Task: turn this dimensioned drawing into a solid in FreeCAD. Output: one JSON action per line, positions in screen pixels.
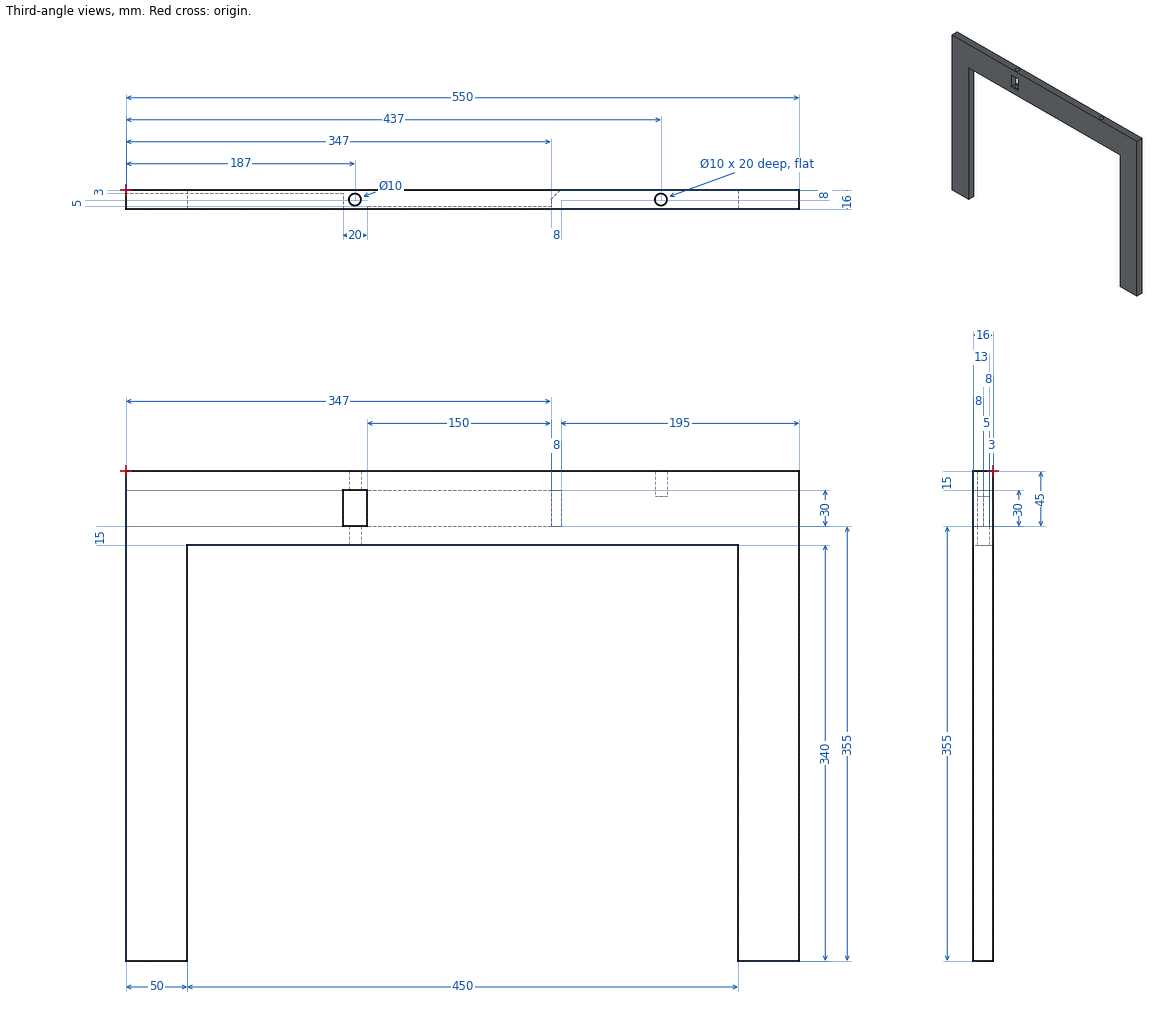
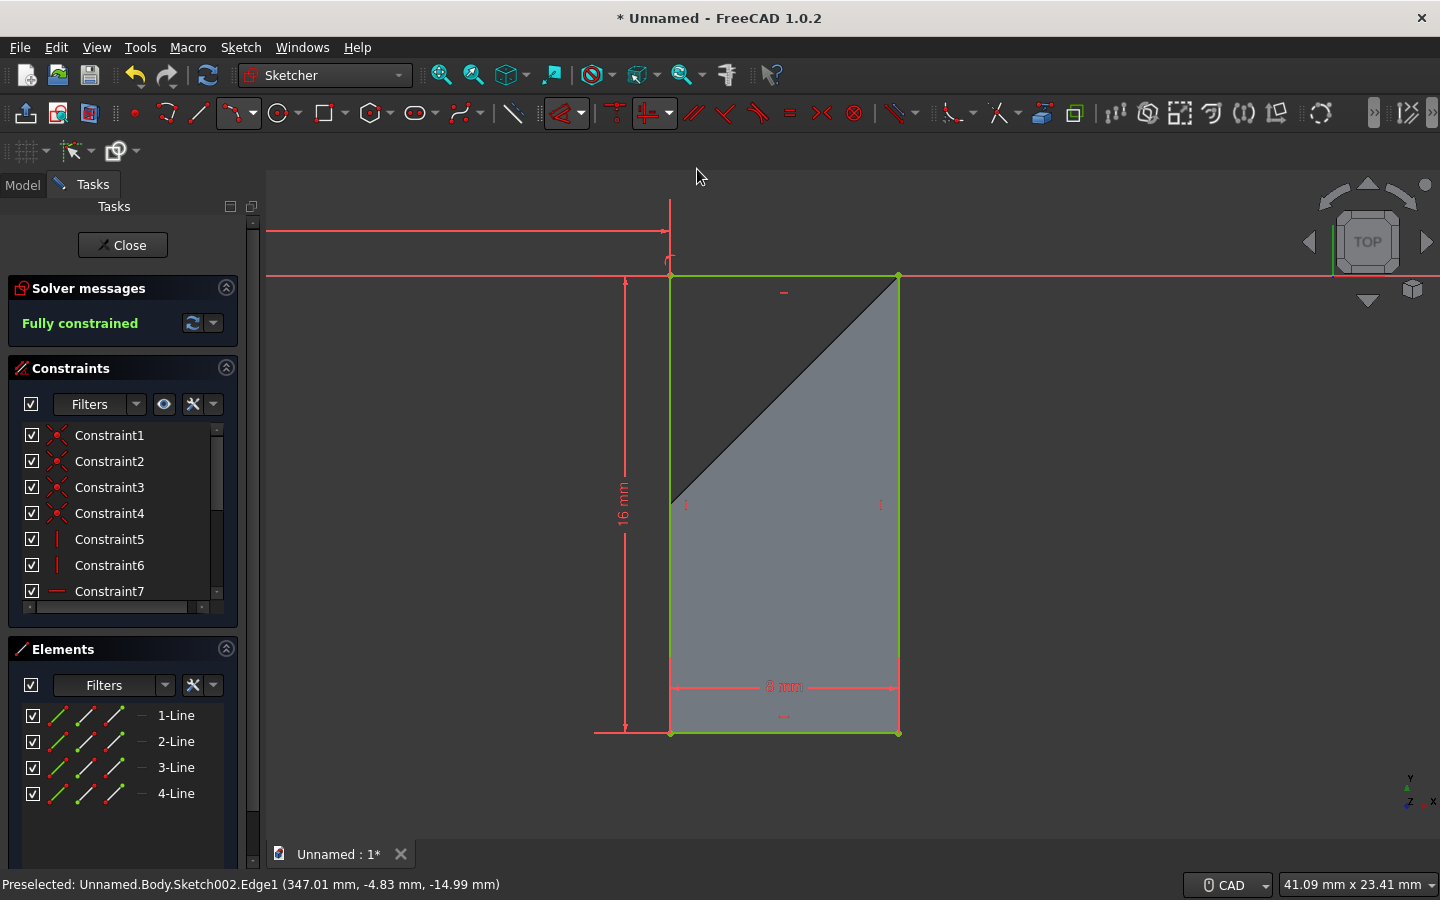
{"action": "left_click", "coordinate": [123, 245]}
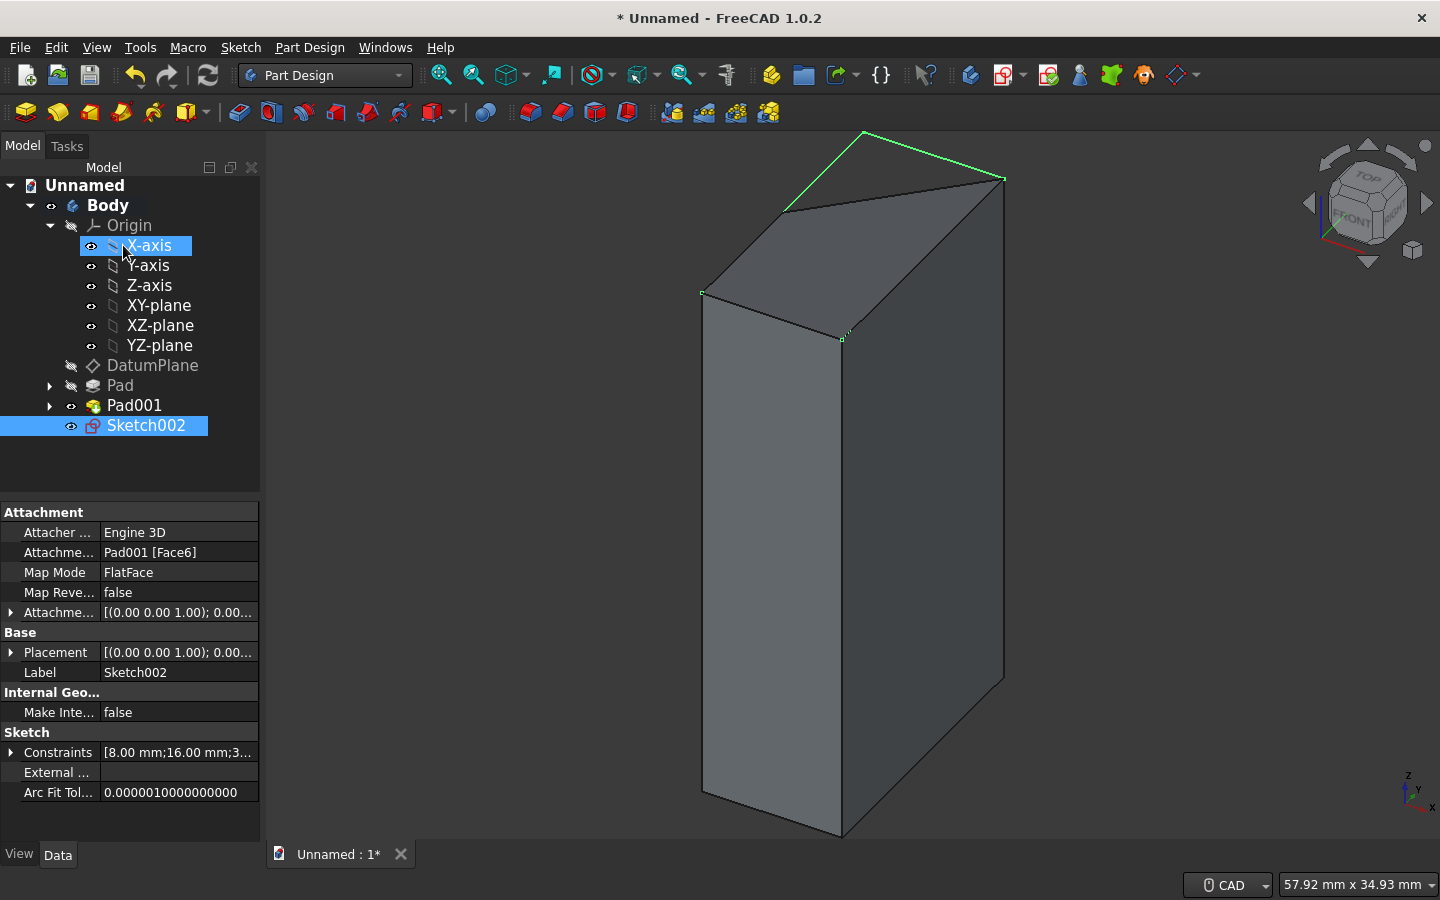
{"action": "left_click", "coordinate": [26, 112]}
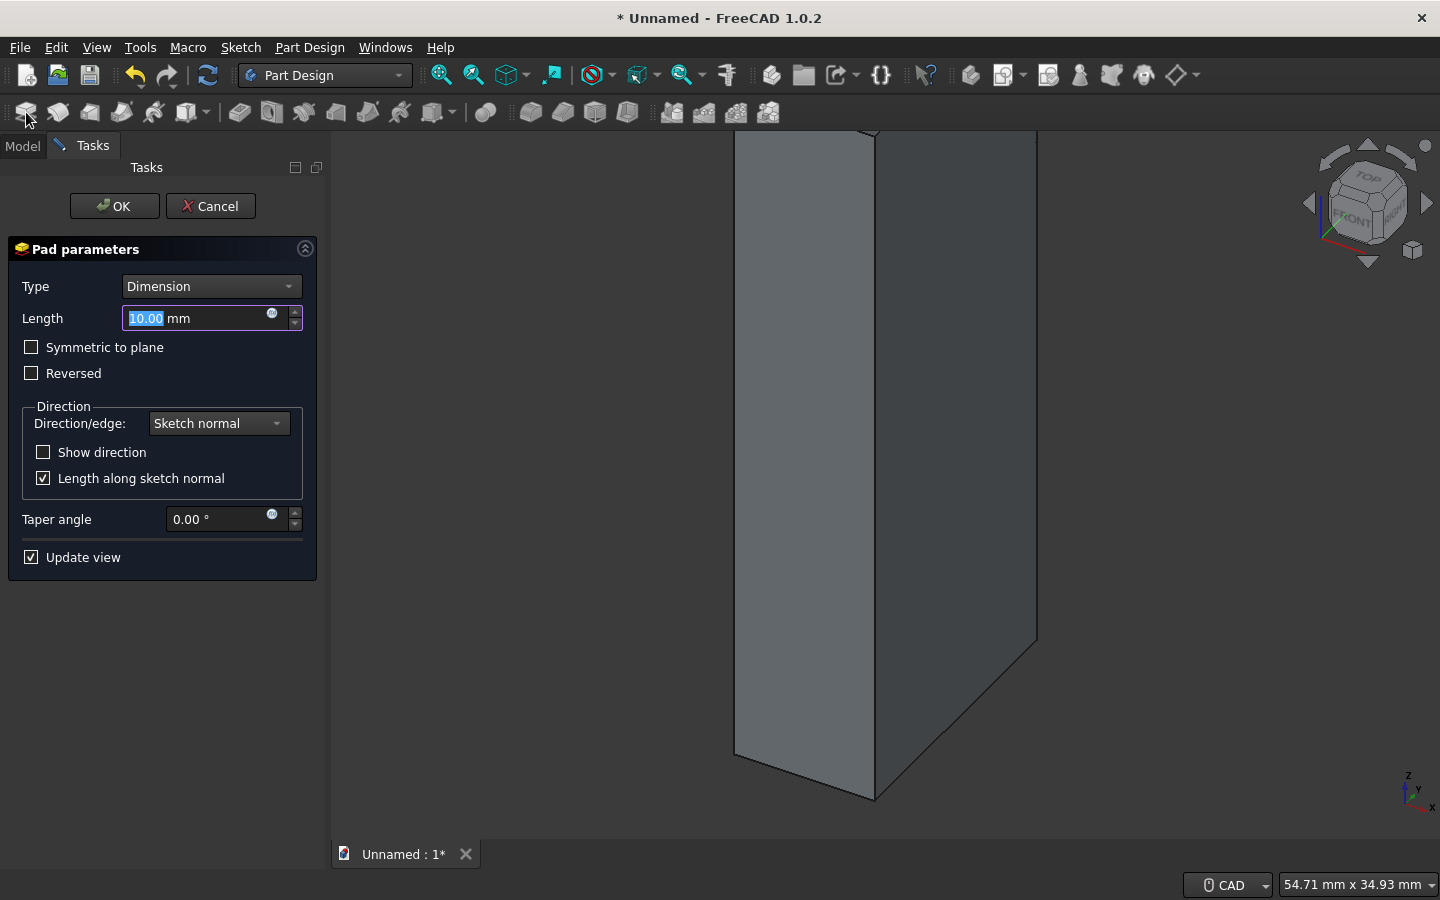
{"action": "type", "text": "15"}
{"action": "key", "text": "Tab"}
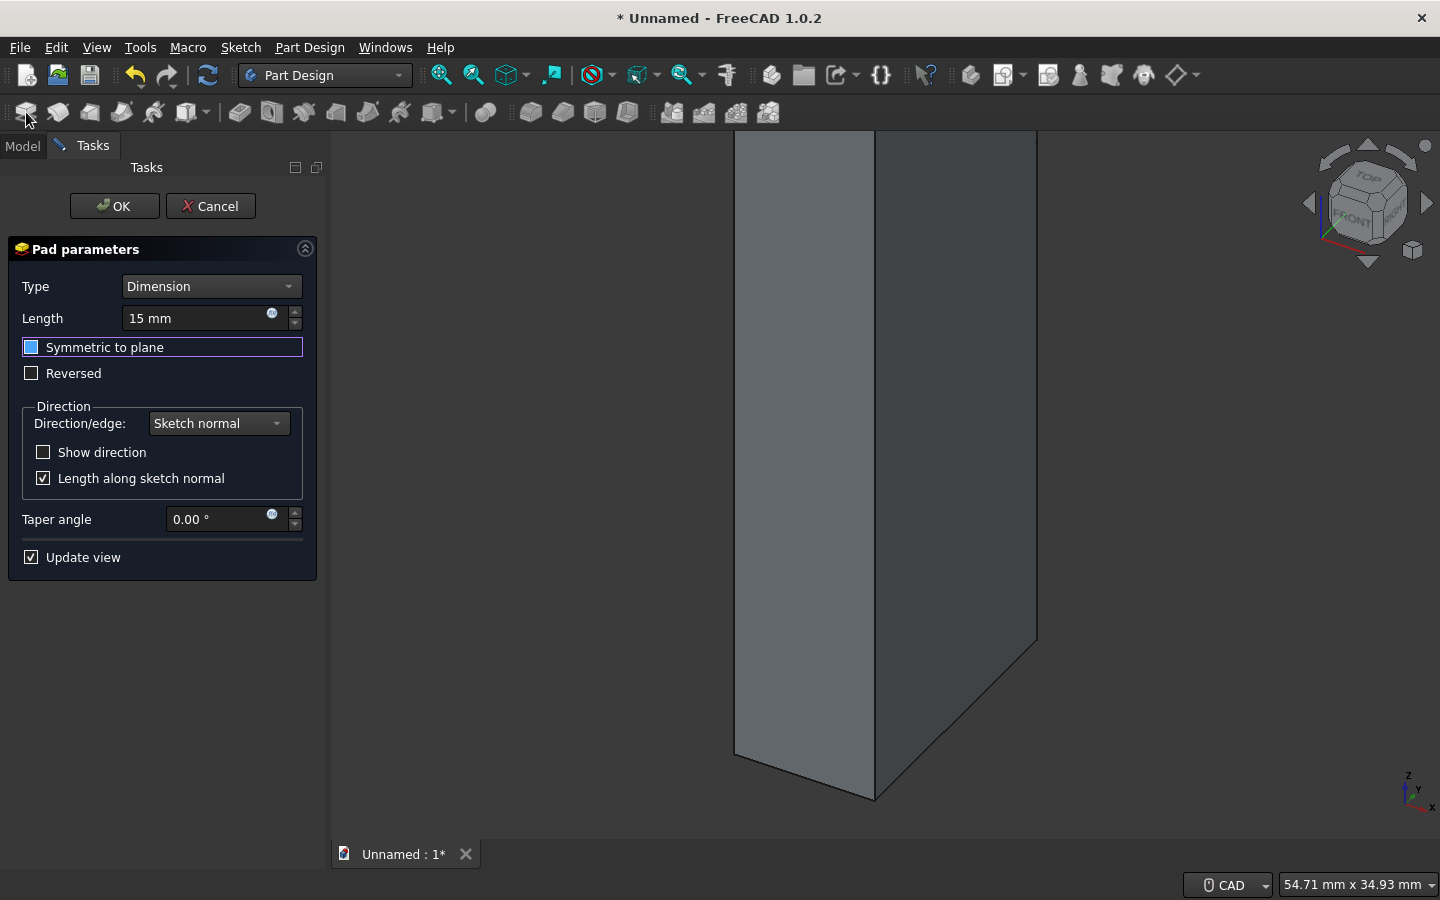
{"action": "left_click", "coordinate": [115, 206]}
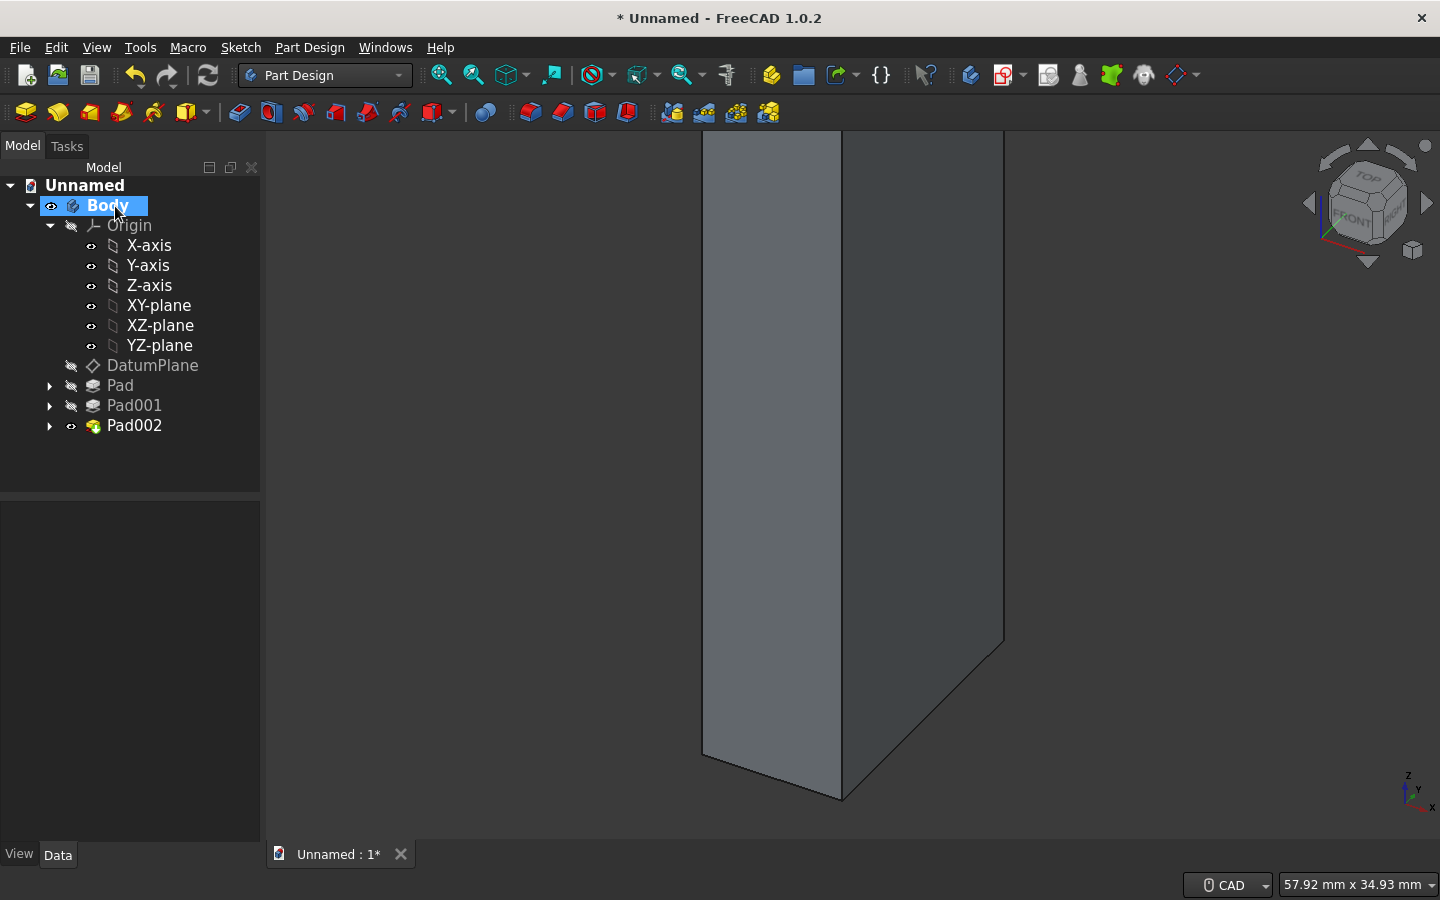
{"action": "left_click", "coordinate": [442, 76]}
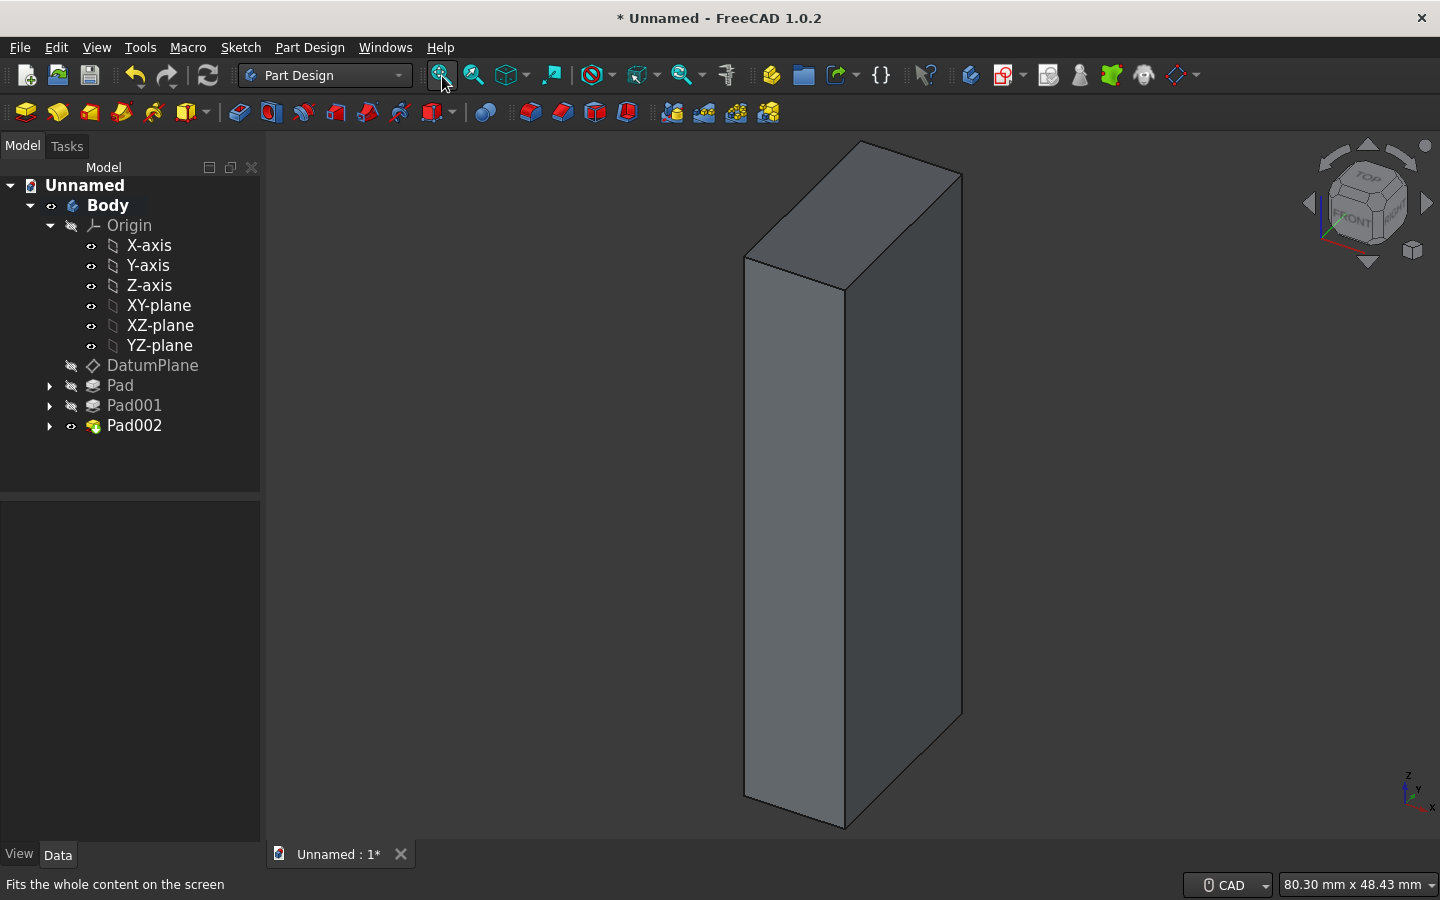
{"action": "left_click", "coordinate": [904, 347]}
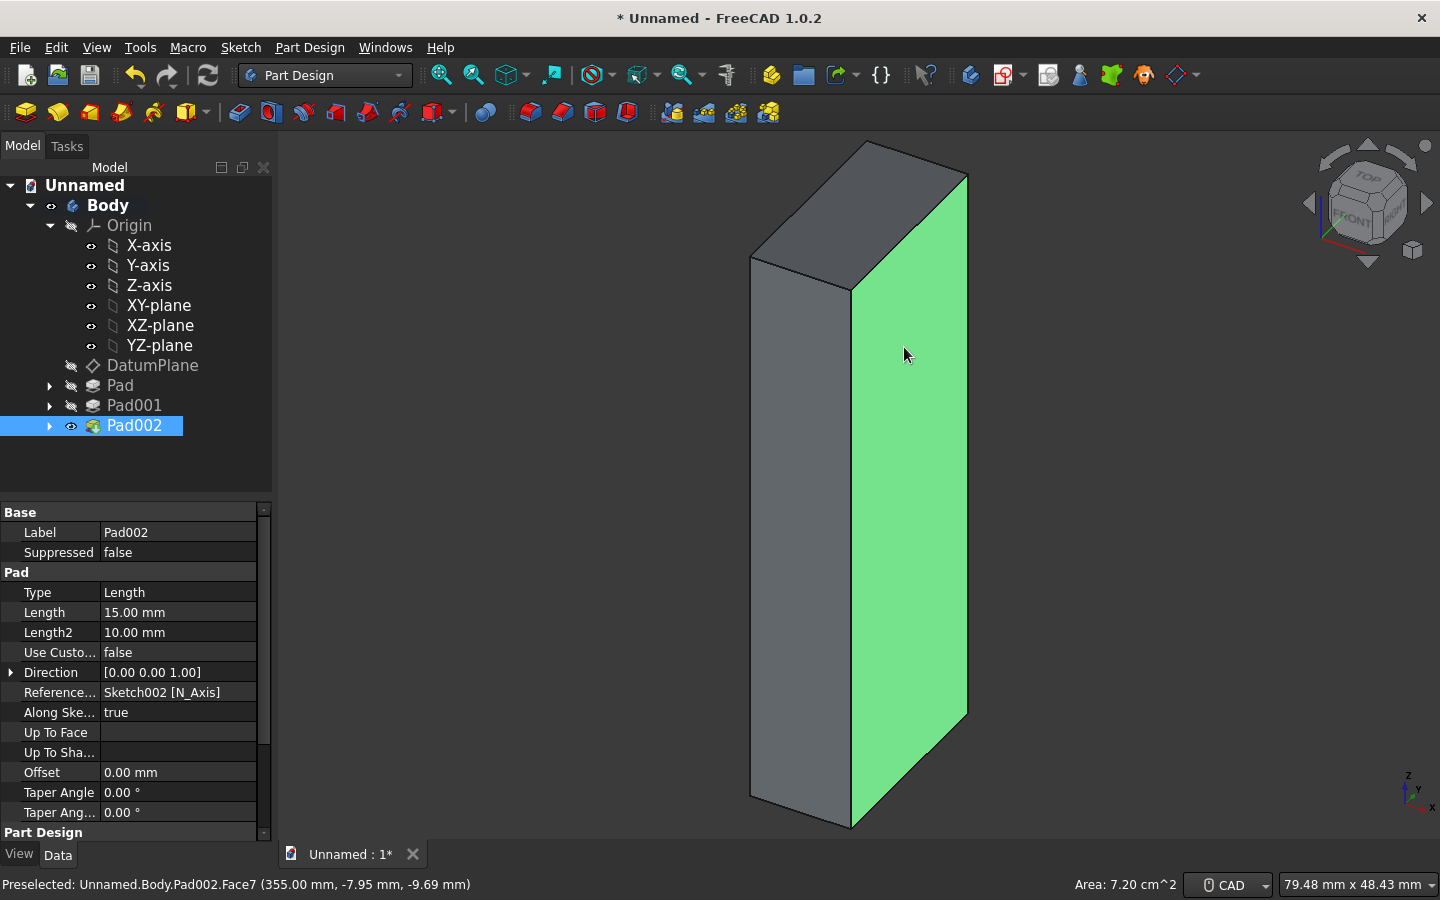
{"action": "left_click", "coordinate": [1004, 76]}